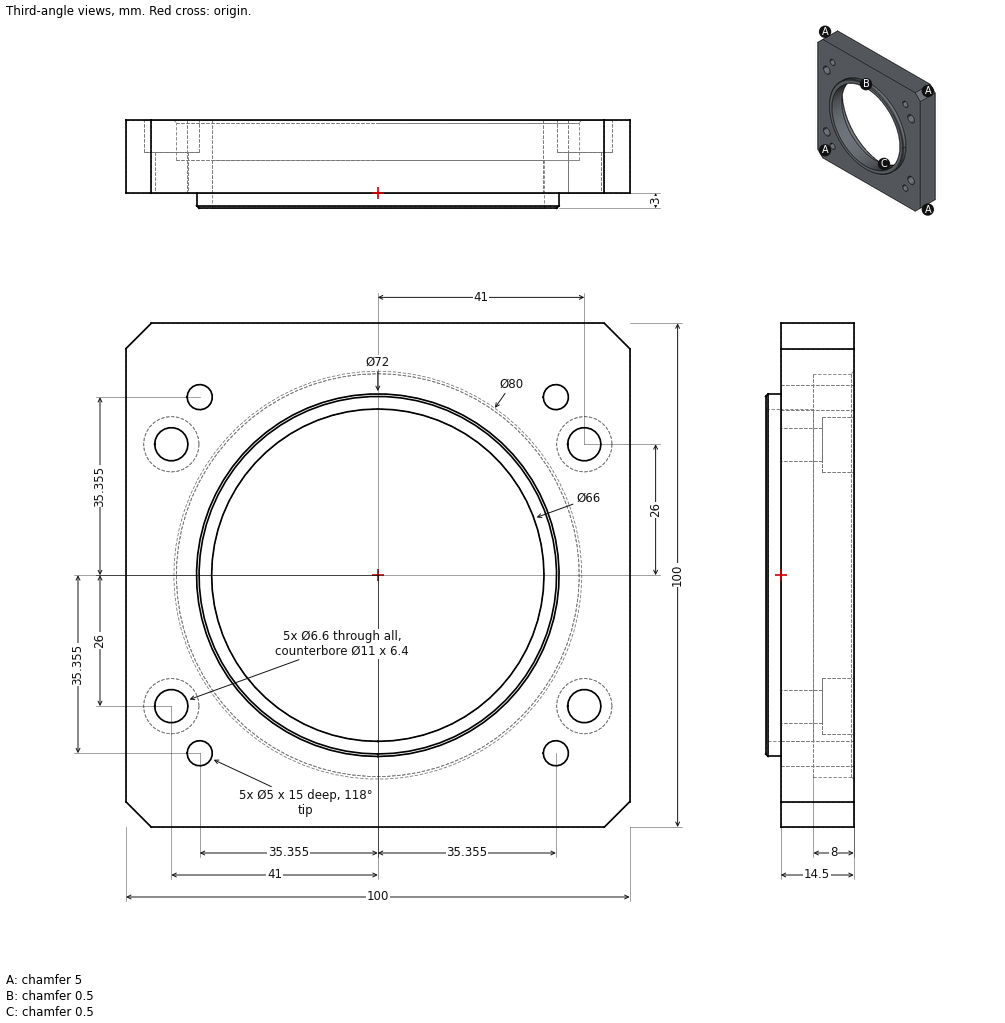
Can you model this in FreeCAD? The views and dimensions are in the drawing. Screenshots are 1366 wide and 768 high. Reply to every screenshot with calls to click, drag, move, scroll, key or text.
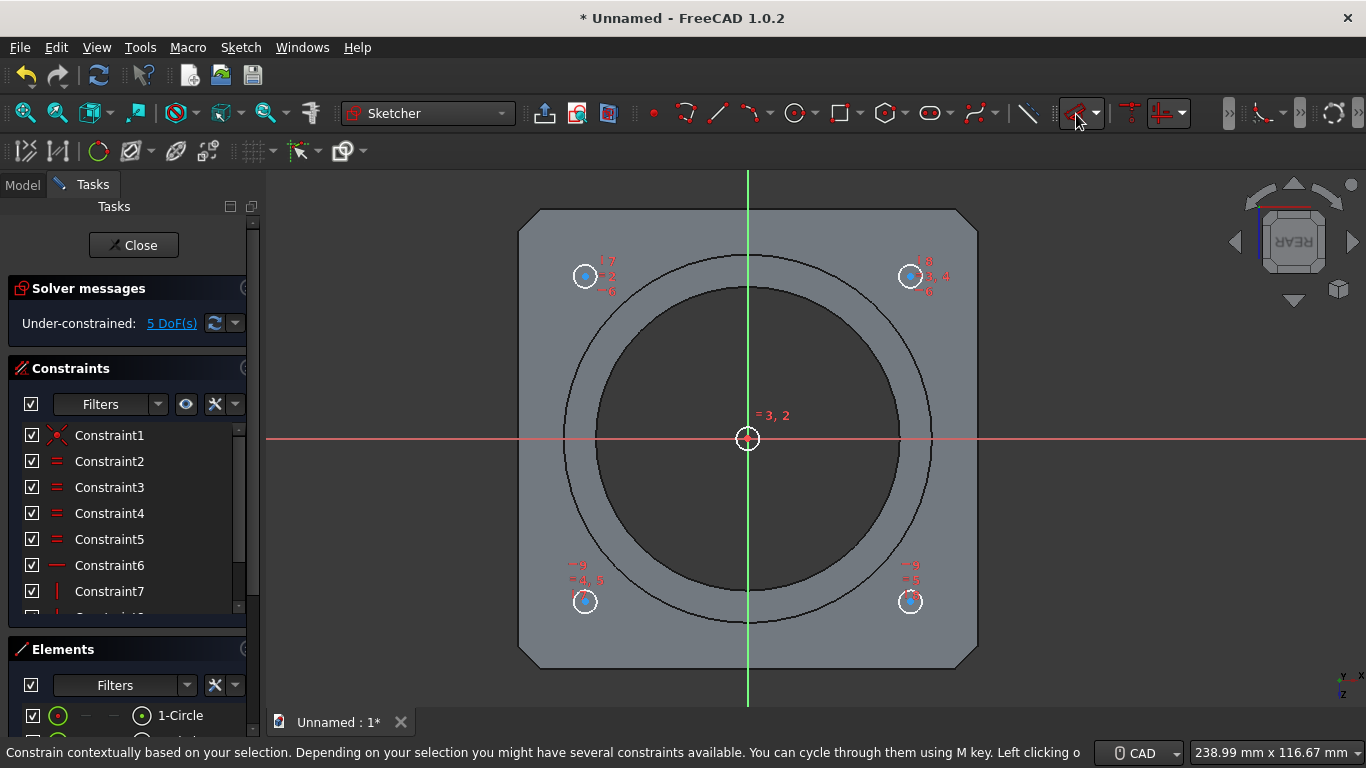
scroll(593, 268, up, 3)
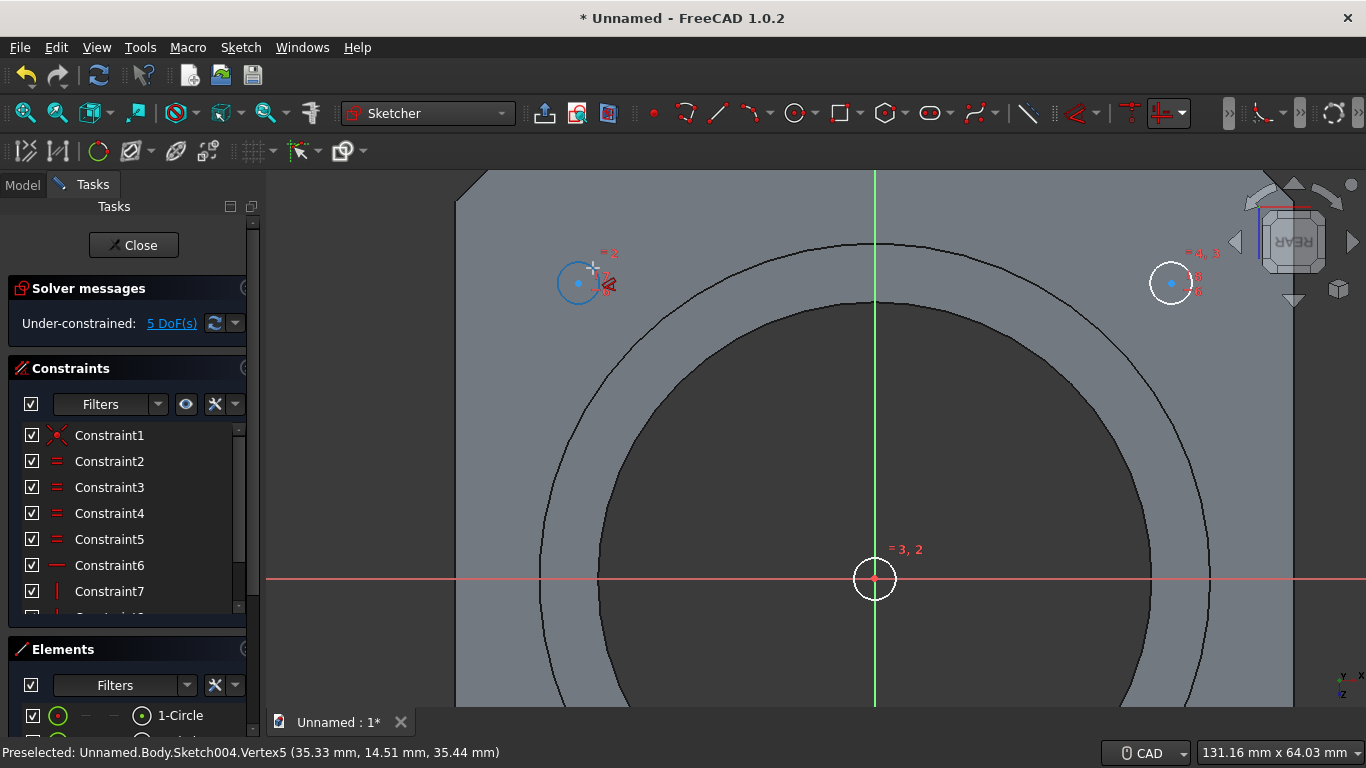
click(593, 268)
click(615, 245)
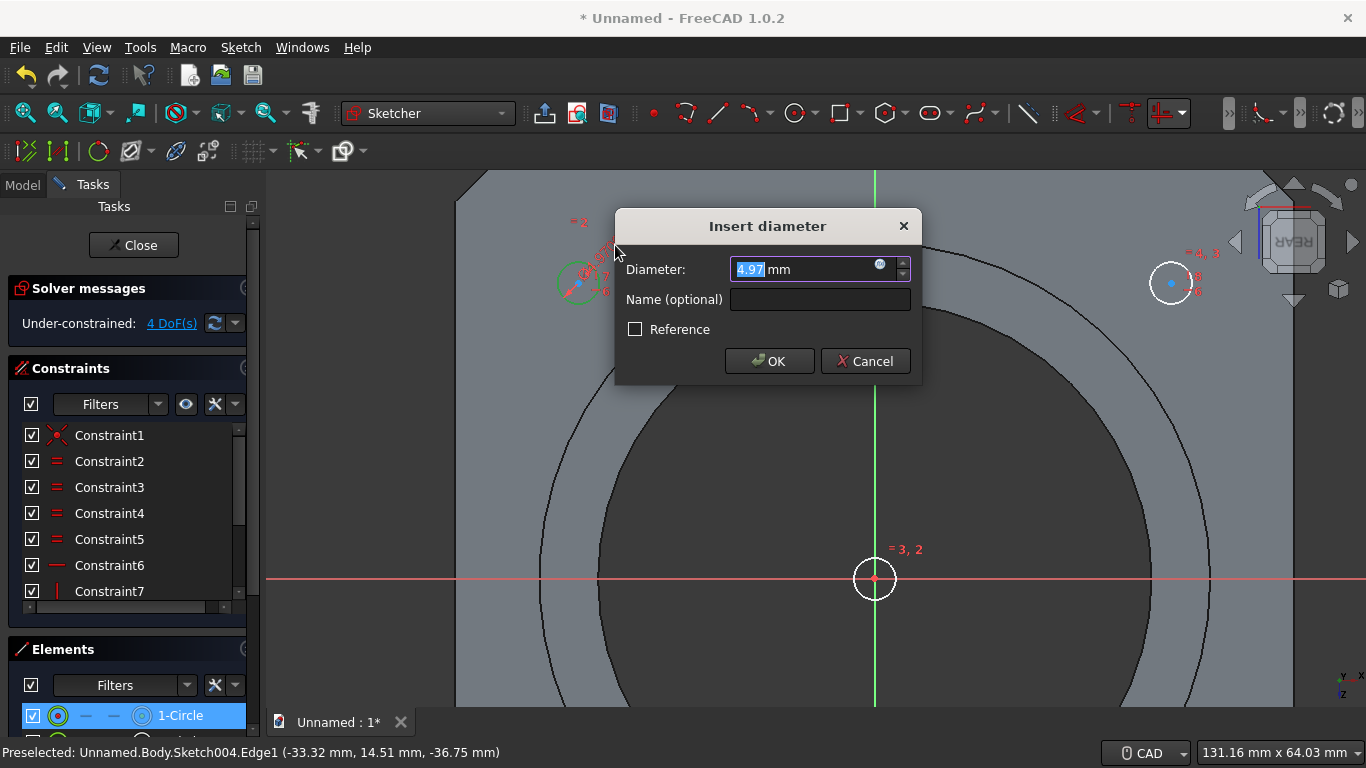
text(5)
key(Return)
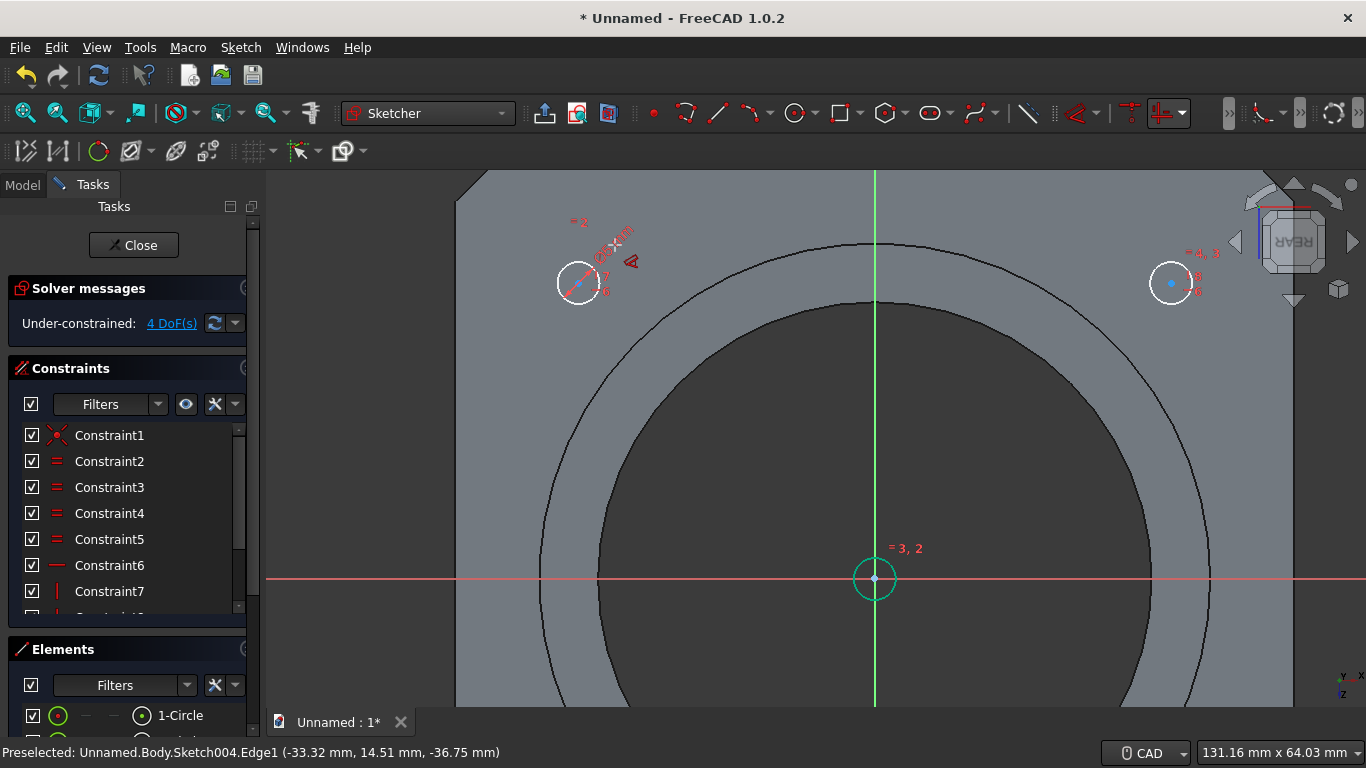
click(579, 283)
click(727, 249)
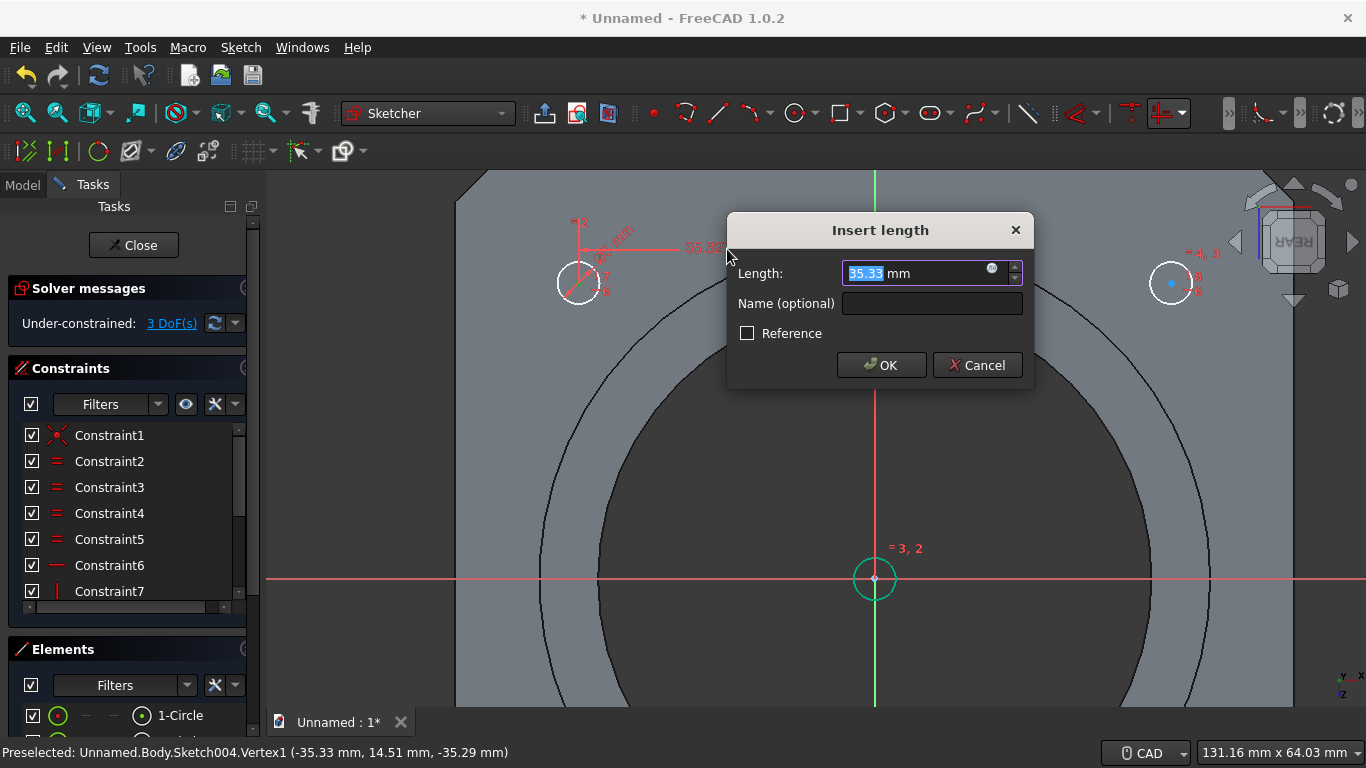
text(35.355)
key(Return)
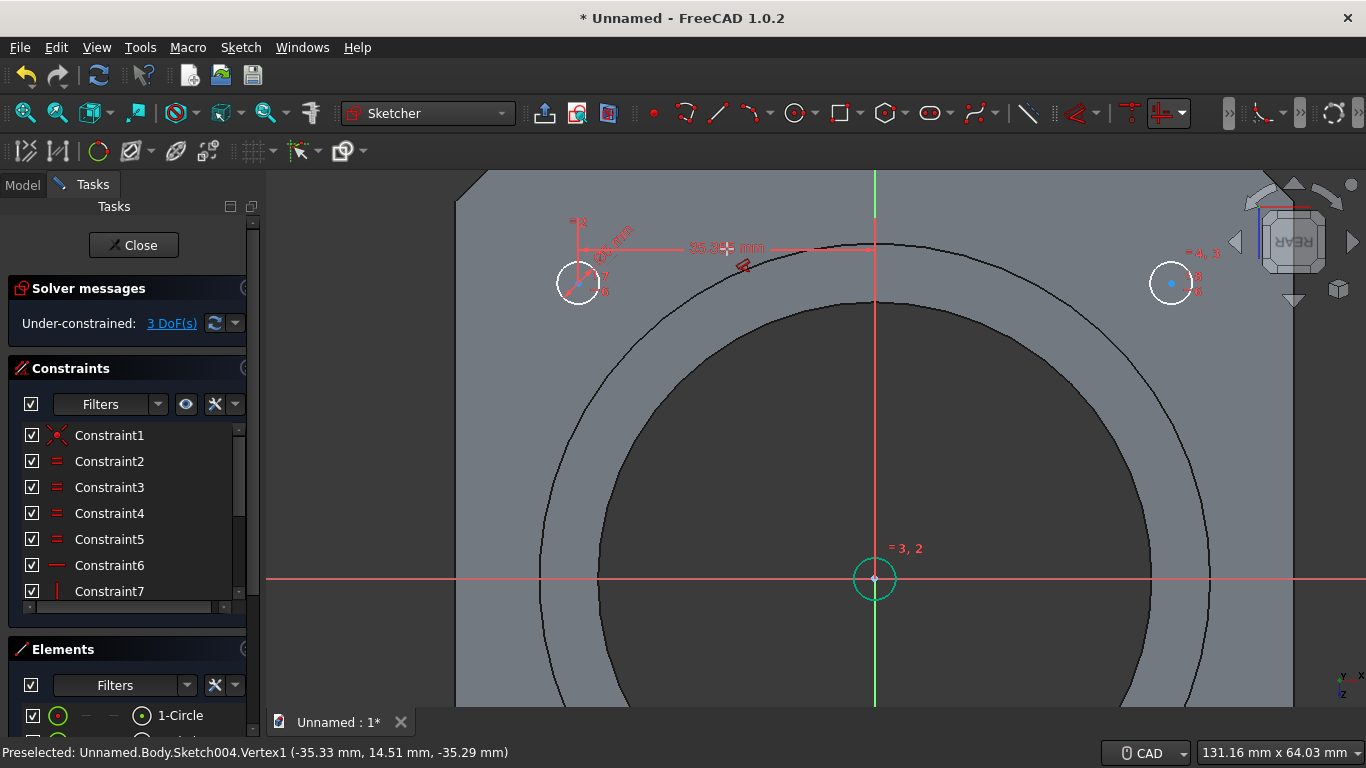
click(578, 283)
click(544, 431)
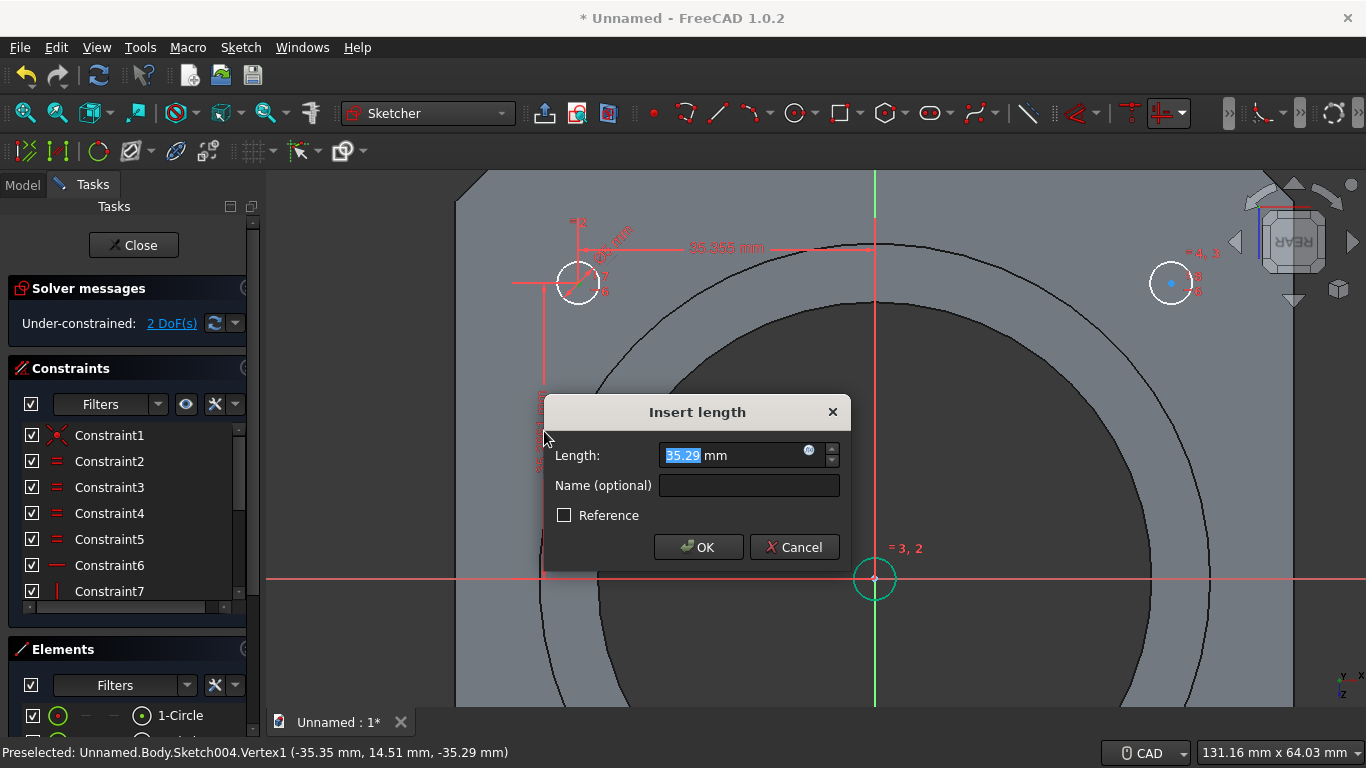
text(35.355)
key(Return)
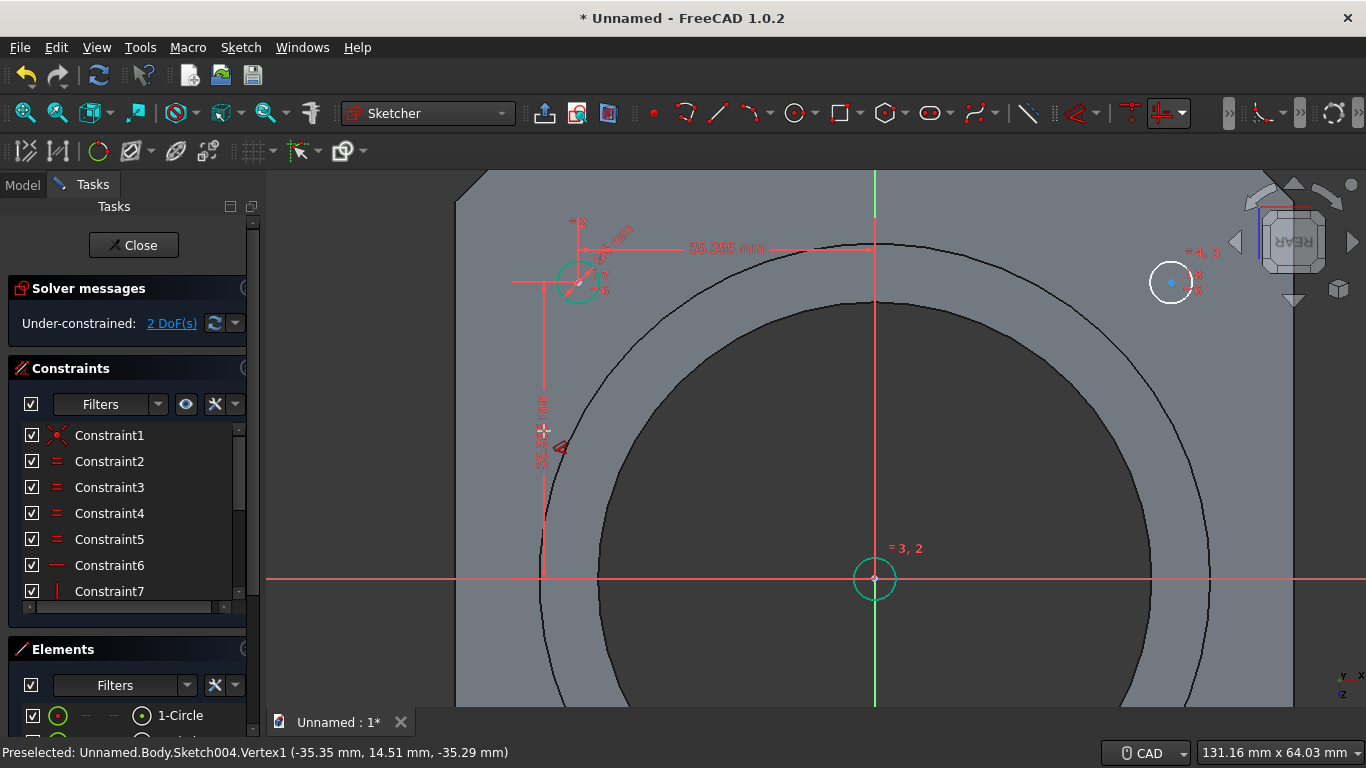
click(1171, 282)
click(1023, 248)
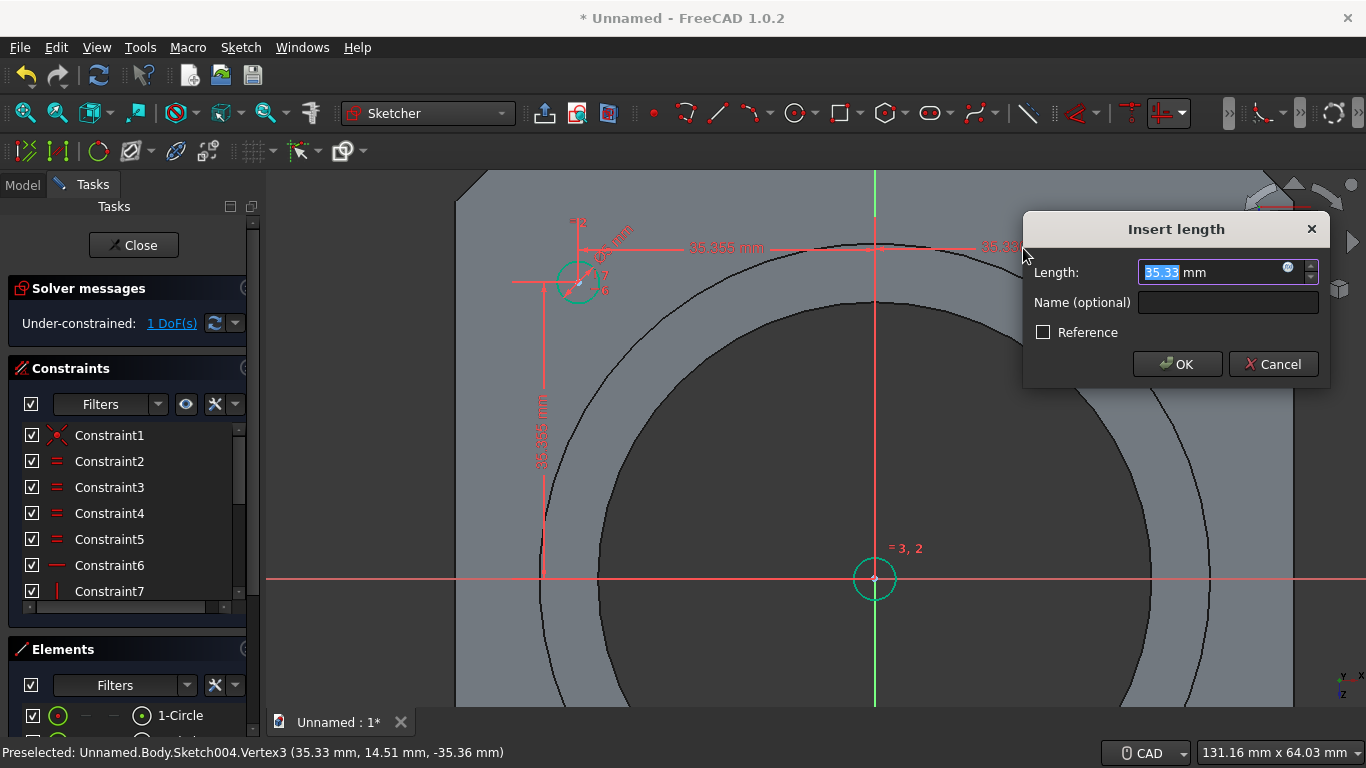
text(35.355)
key(Return)